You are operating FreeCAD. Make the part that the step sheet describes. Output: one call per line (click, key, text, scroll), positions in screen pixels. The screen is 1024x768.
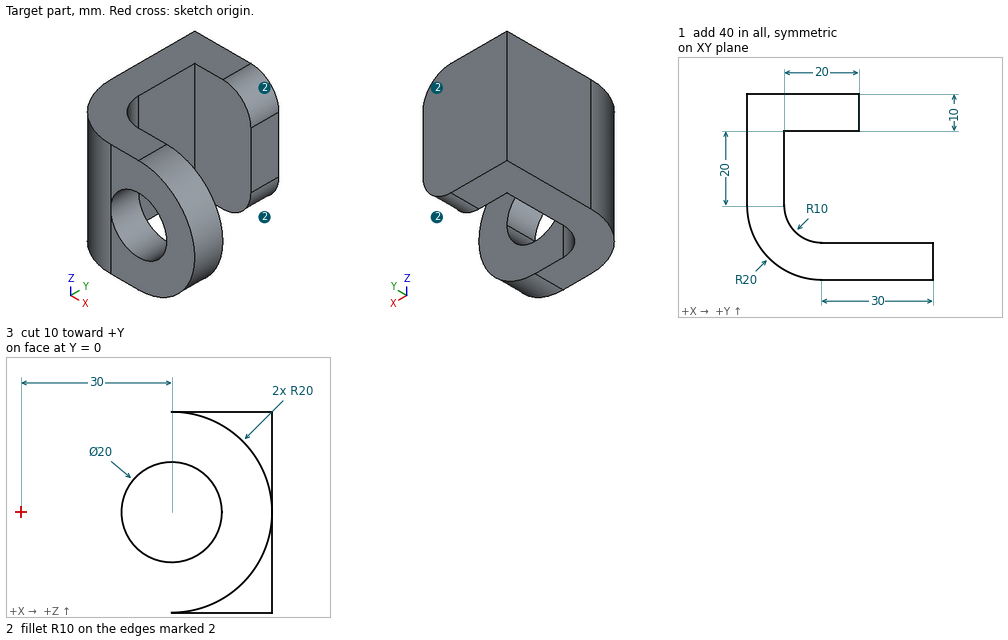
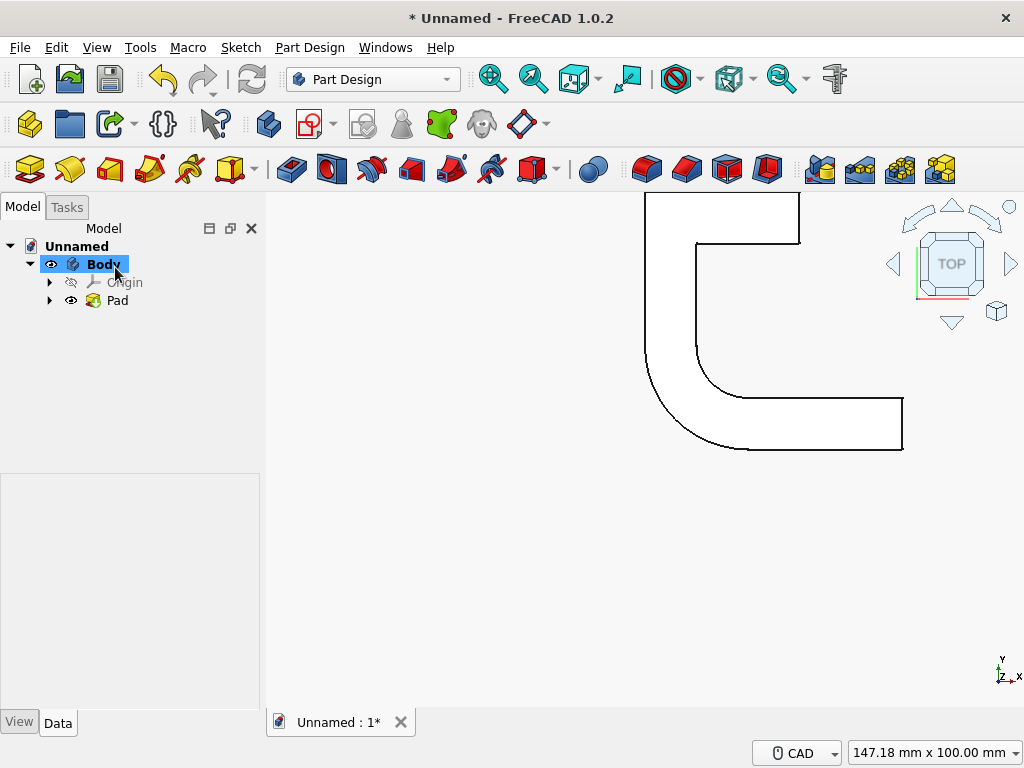
click(494, 80)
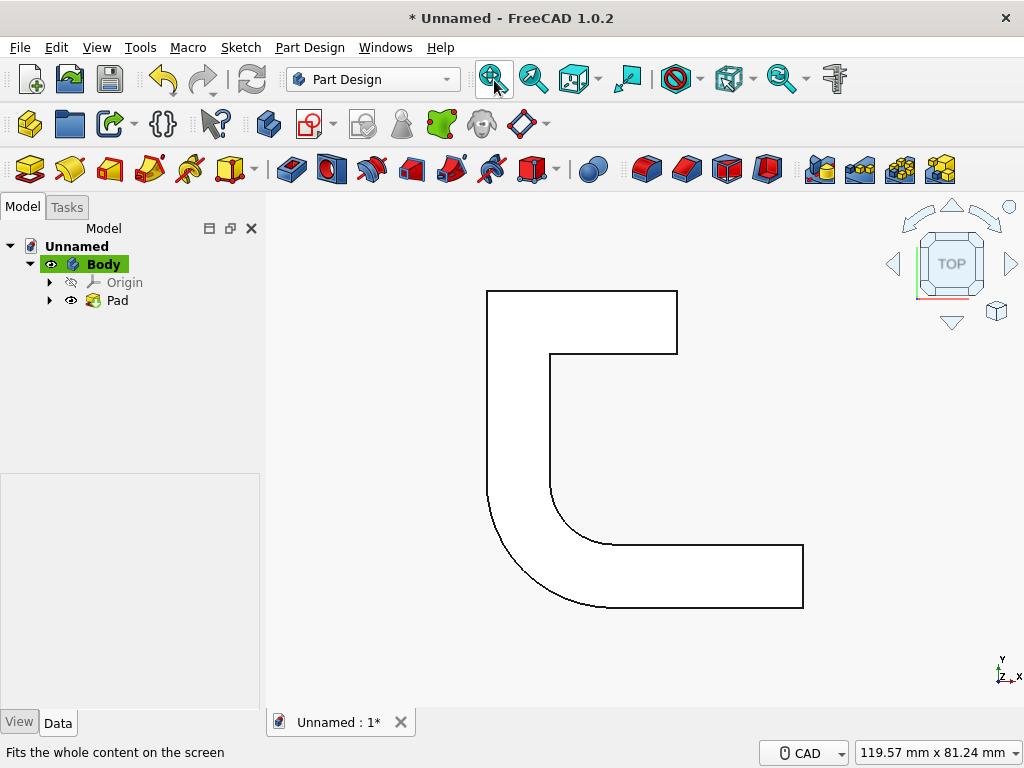
click(677, 322)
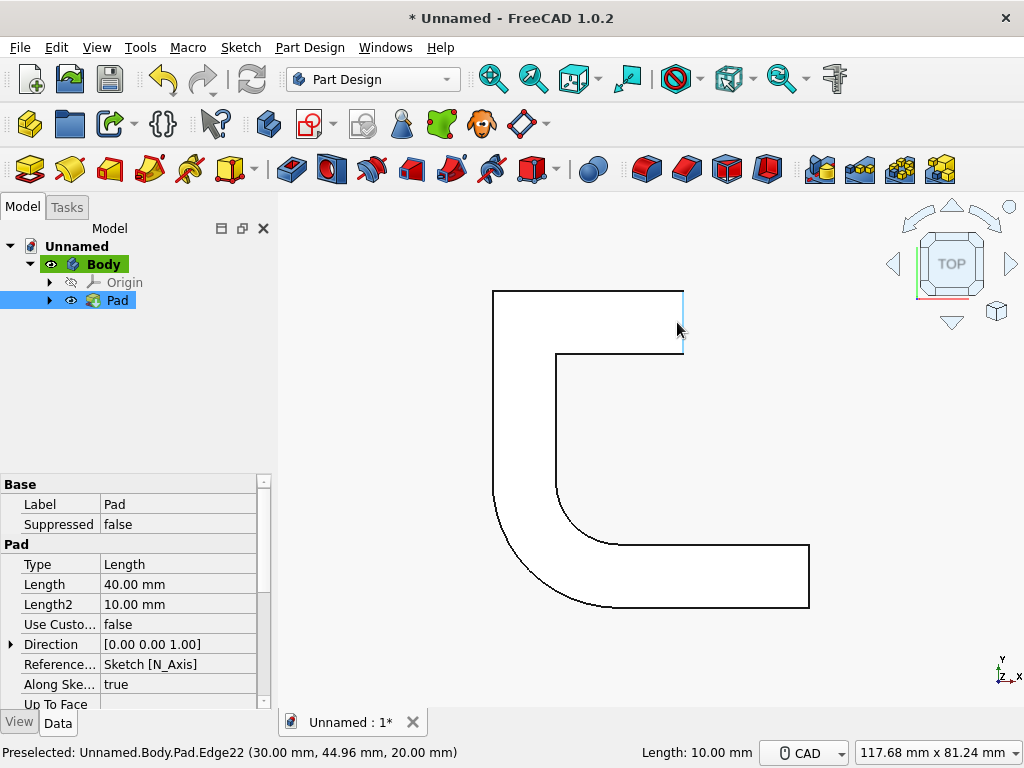
key(1)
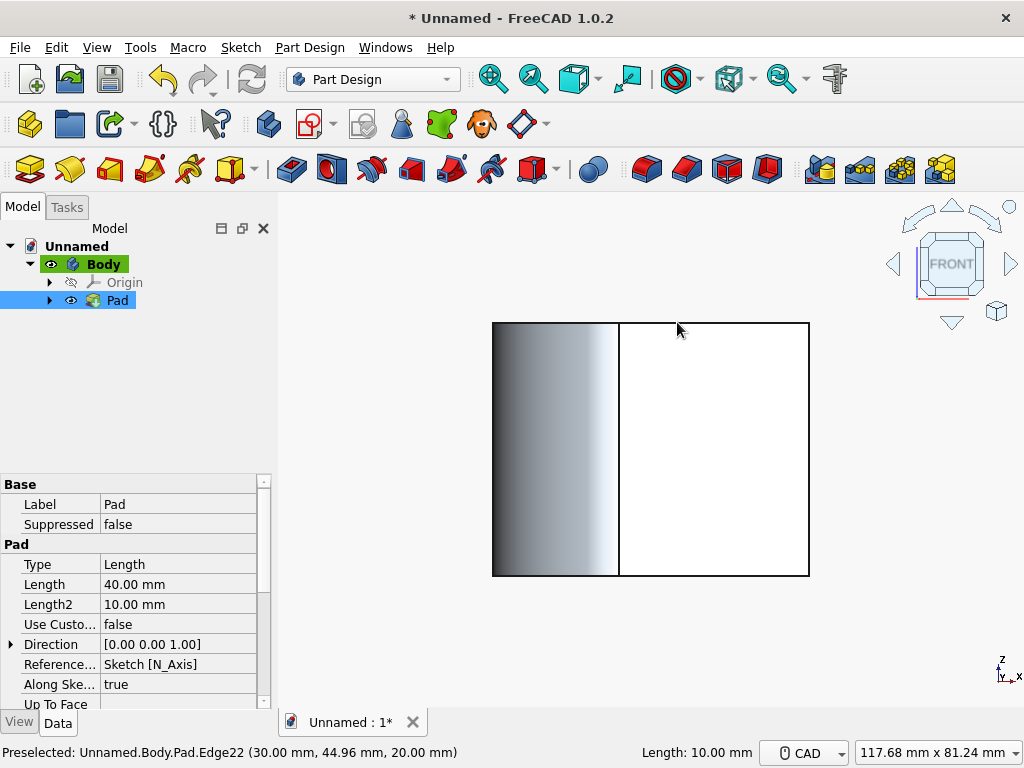
key(3)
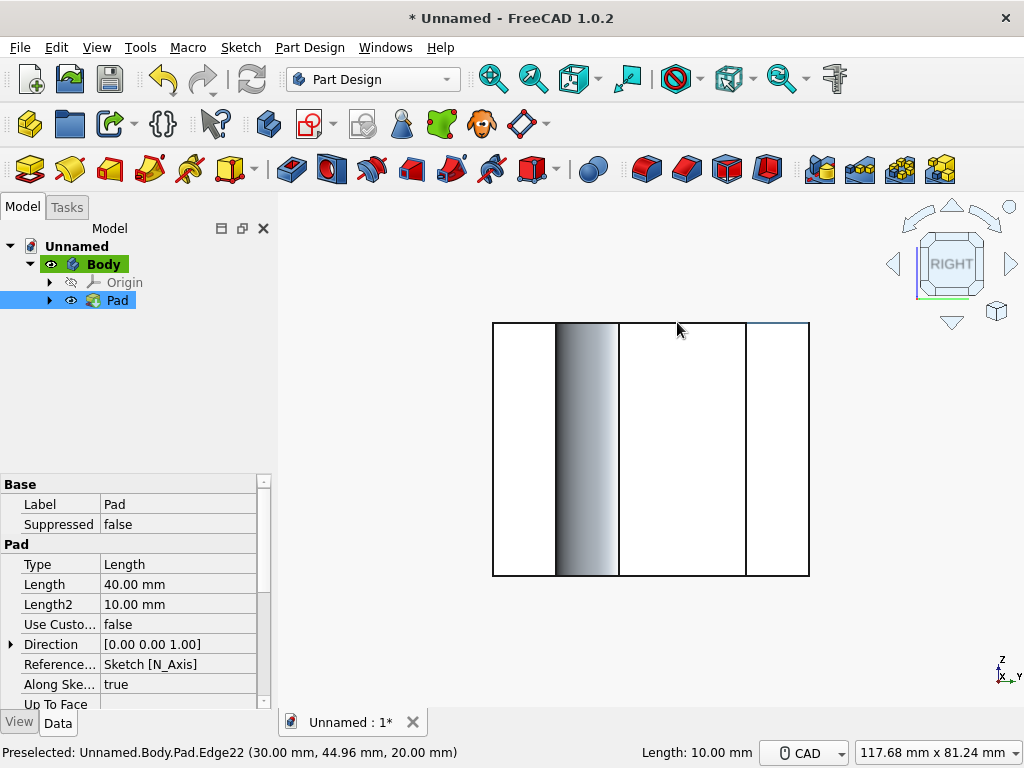
click(778, 575, ctrl)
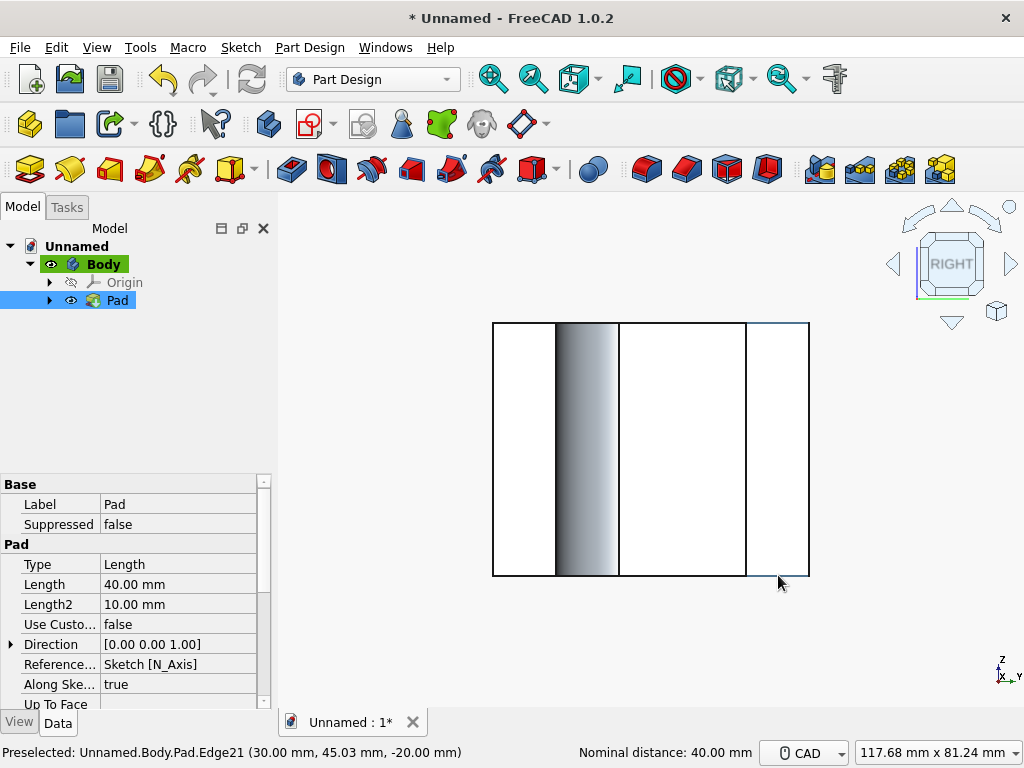
click(648, 170)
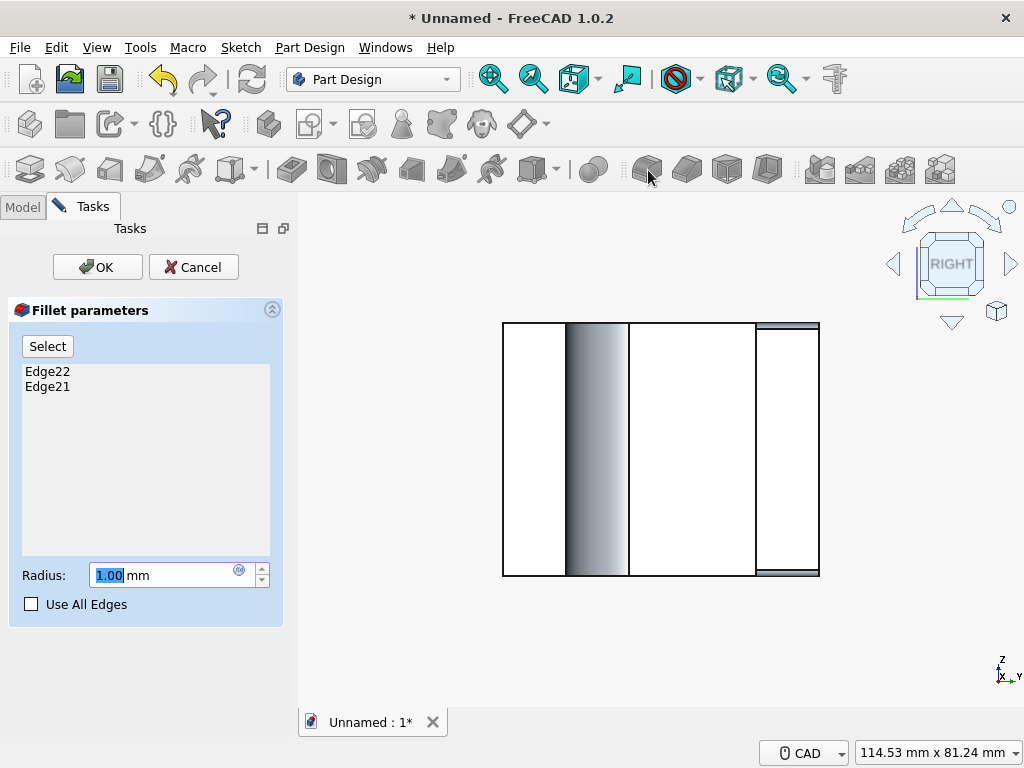
text(10)
key(Tab)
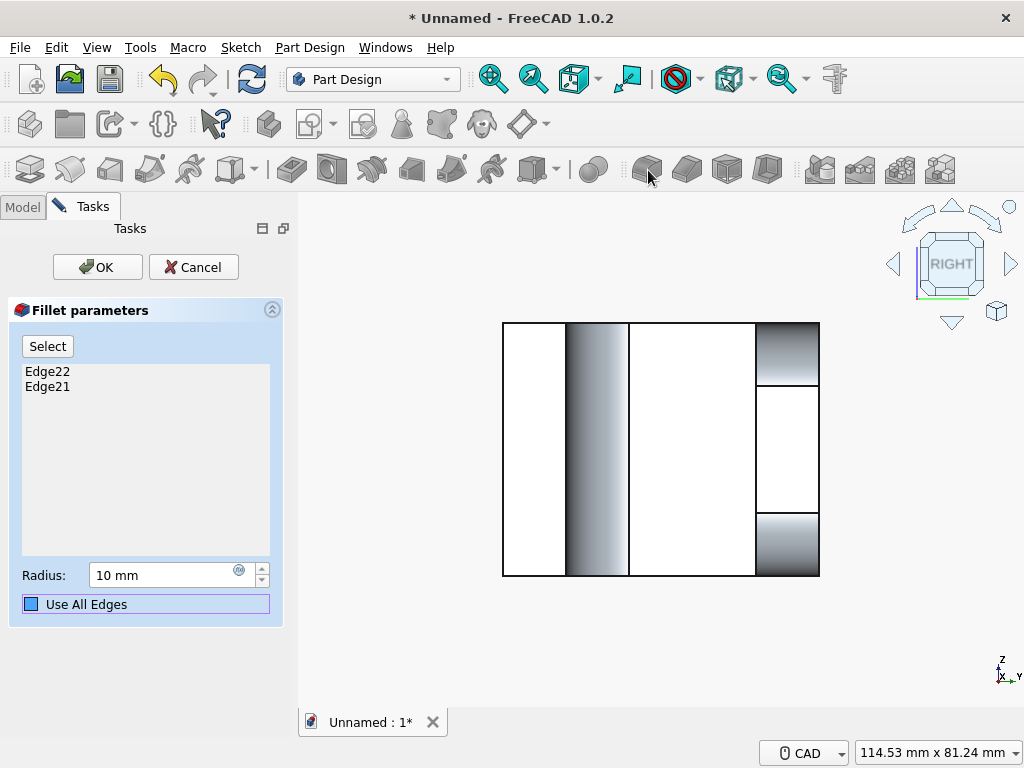
click(98, 267)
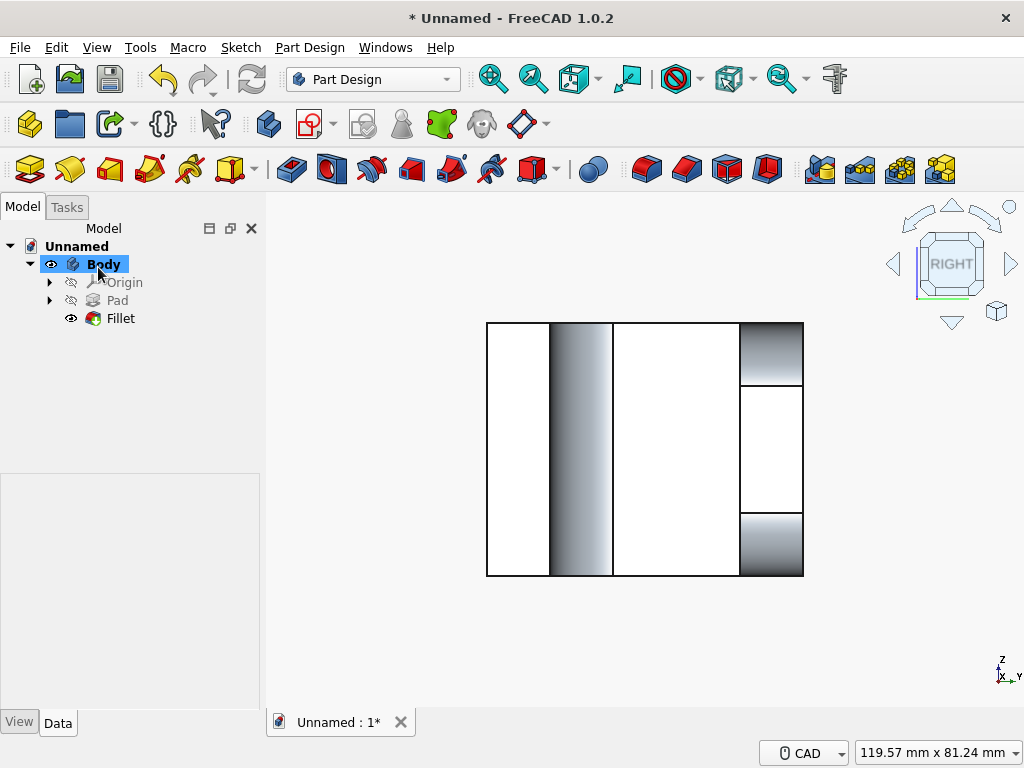
key(0)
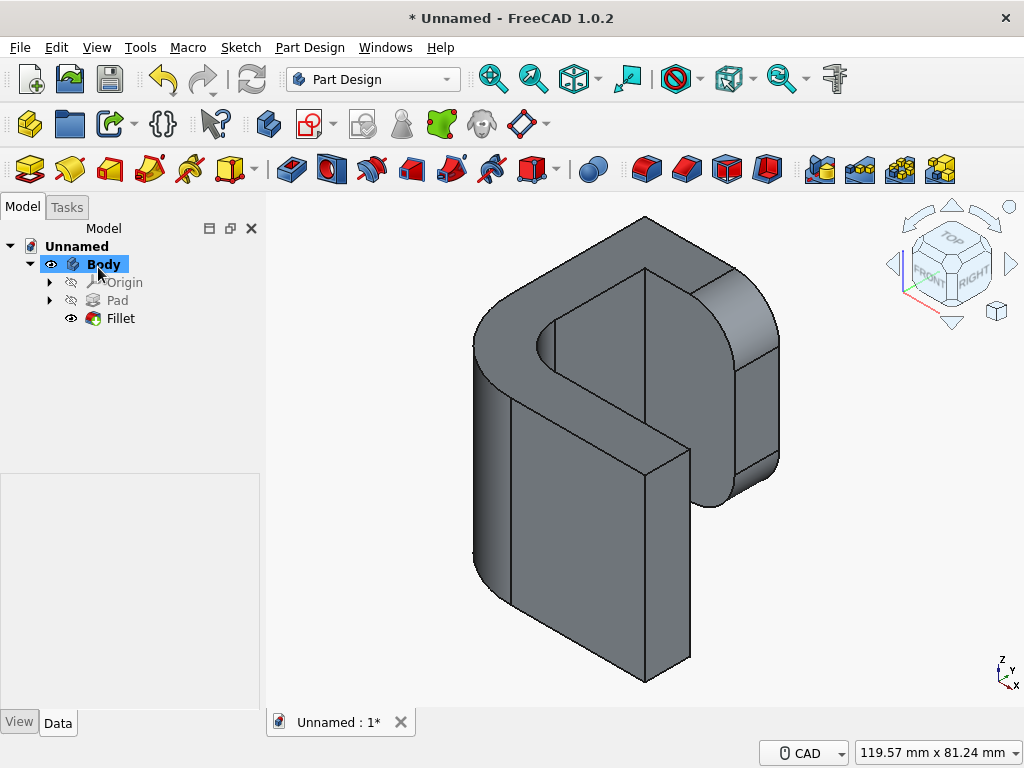
click(578, 539)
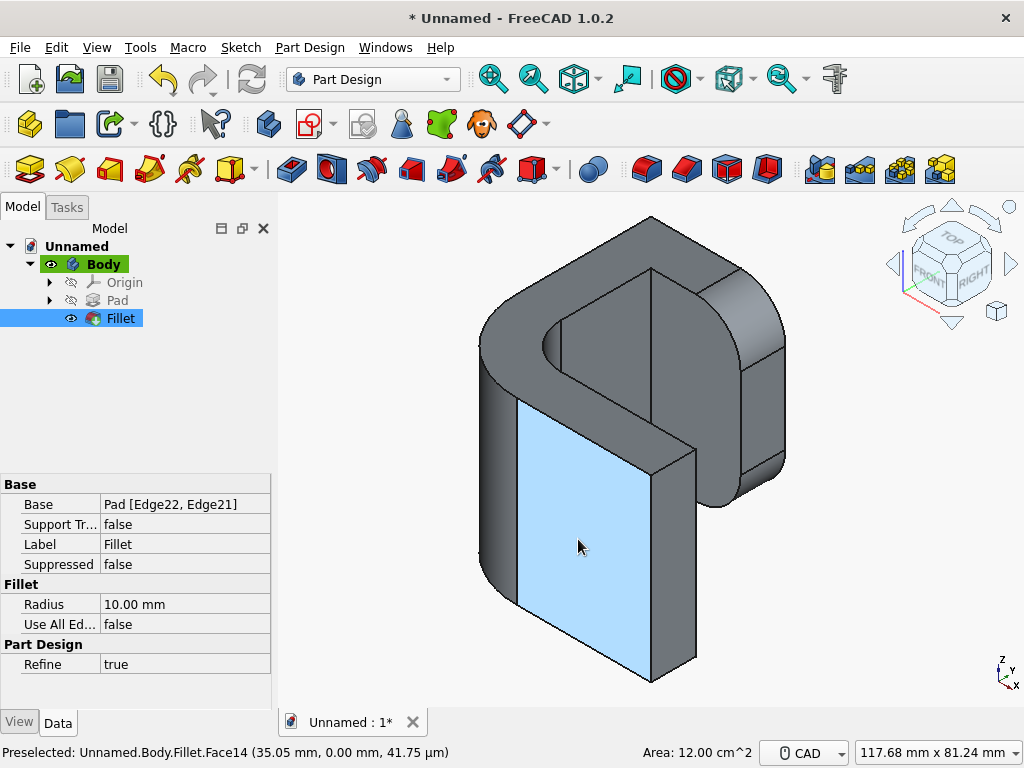
click(310, 124)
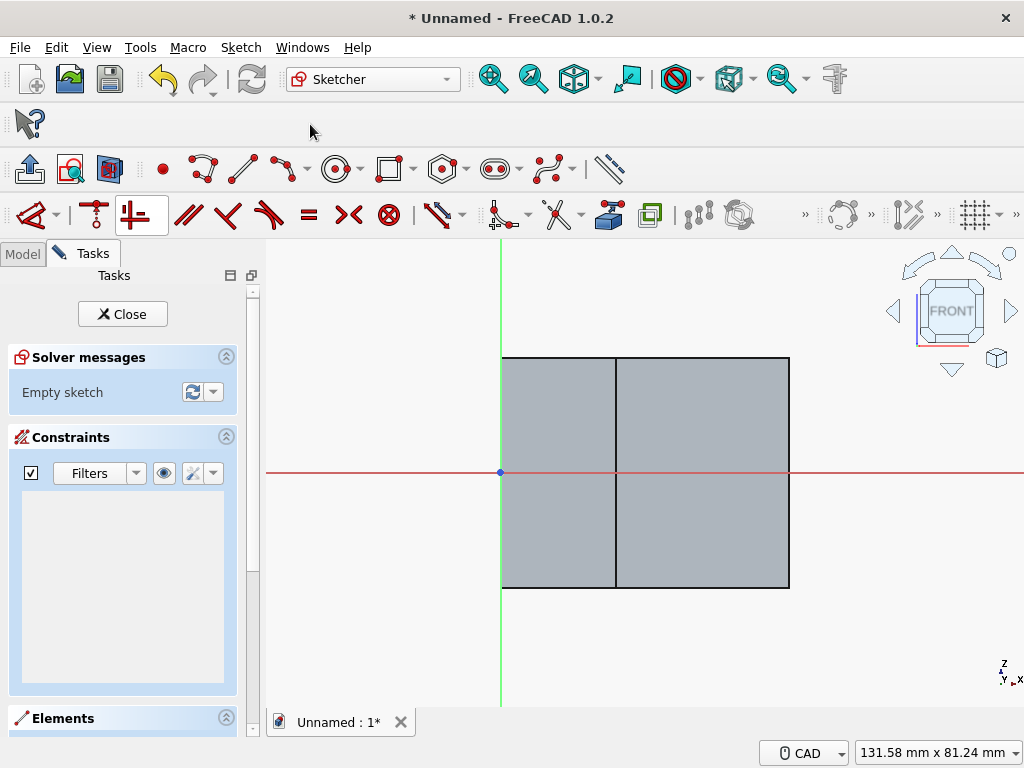
key(g)
key(m)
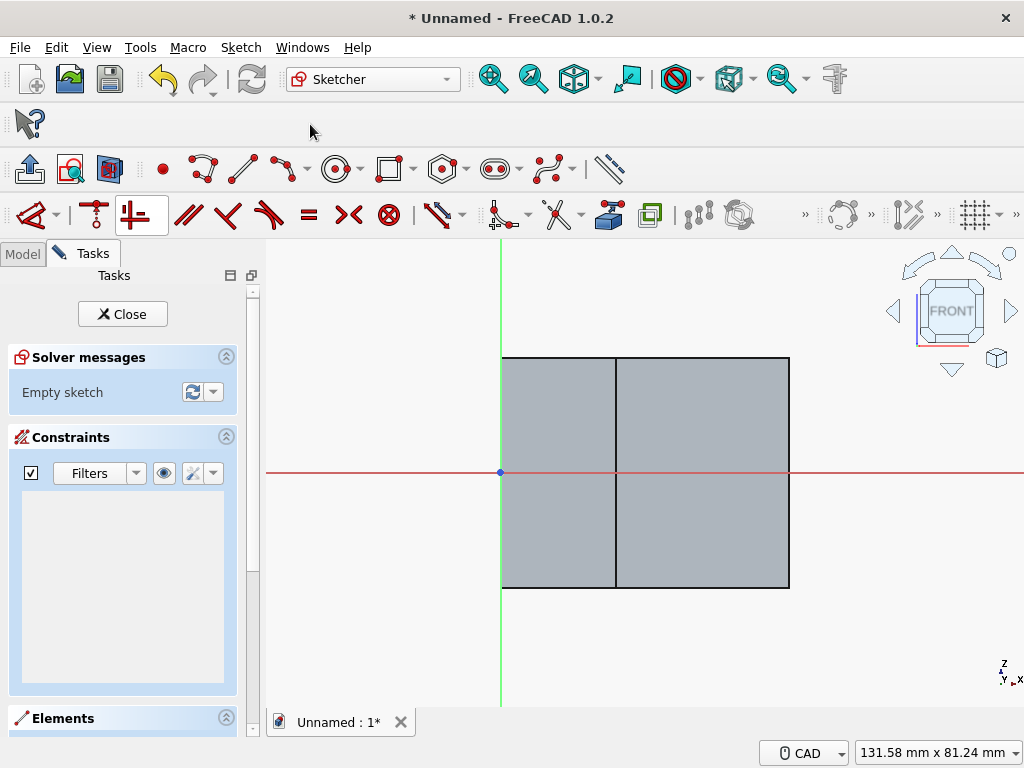
click(789, 473)
click(789, 358)
click(674, 358)
right_click(674, 358)